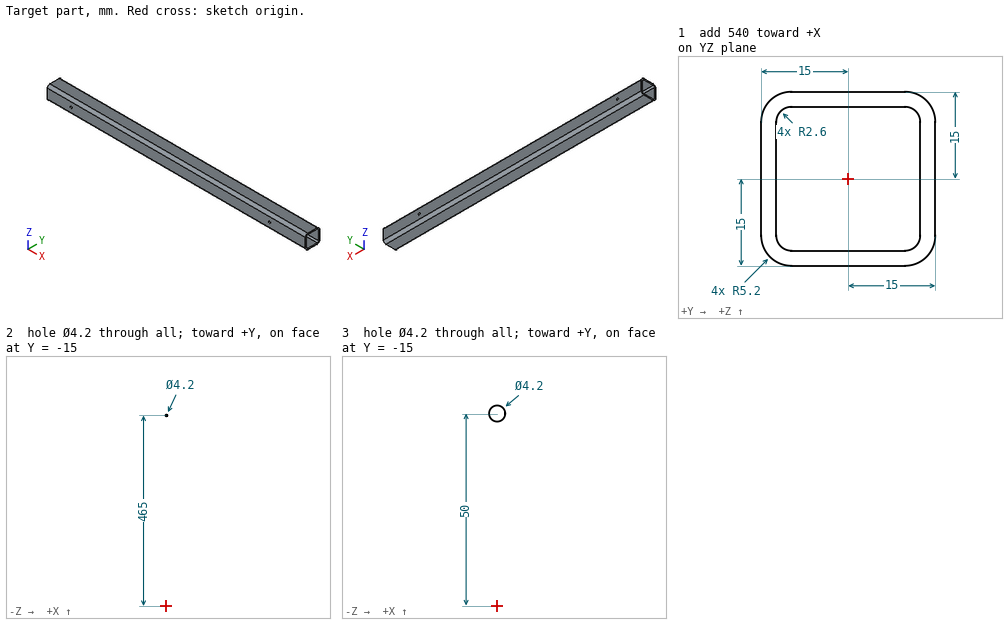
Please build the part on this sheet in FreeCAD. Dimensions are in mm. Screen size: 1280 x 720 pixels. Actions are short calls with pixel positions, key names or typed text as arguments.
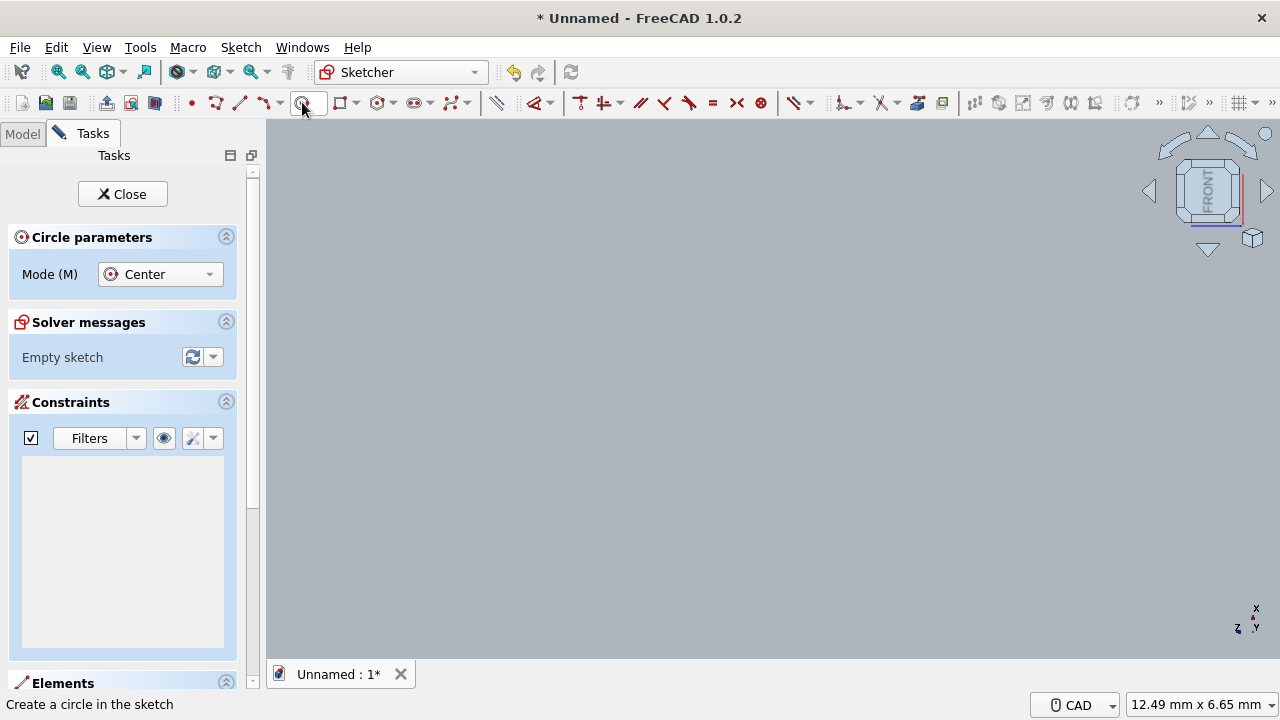
click(704, 388)
click(825, 268)
key(Escape)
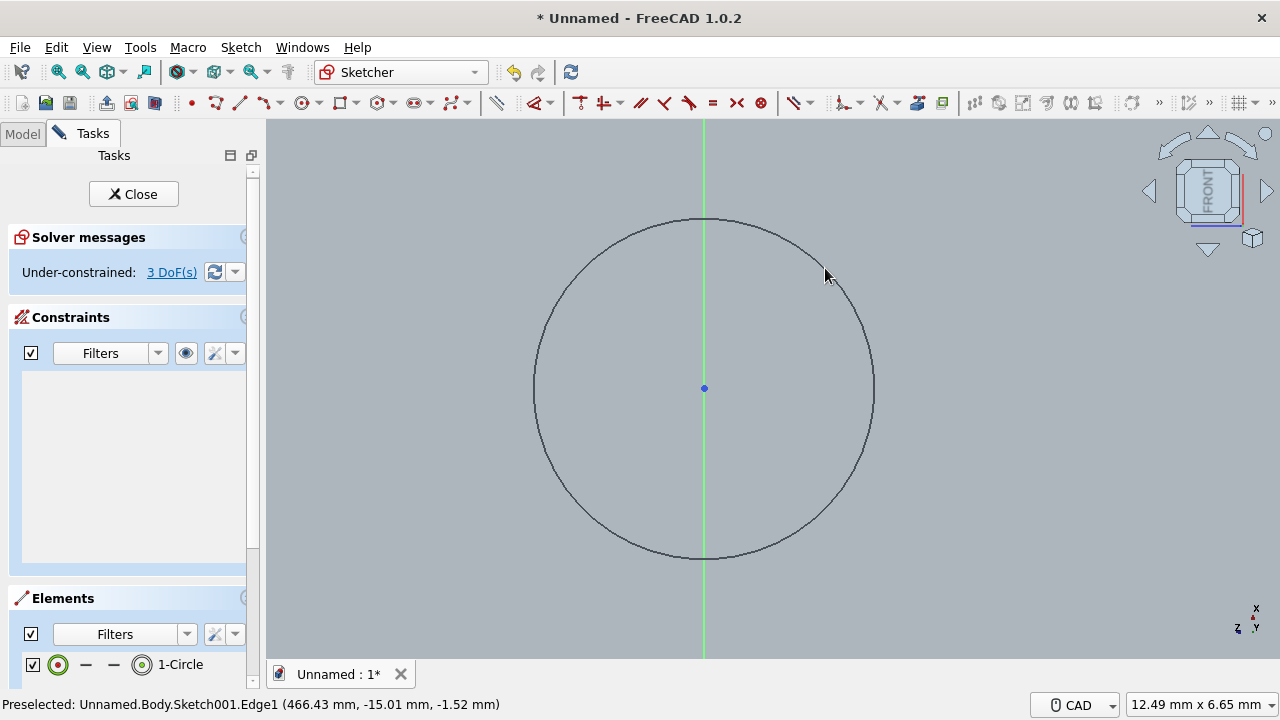
click(704, 389)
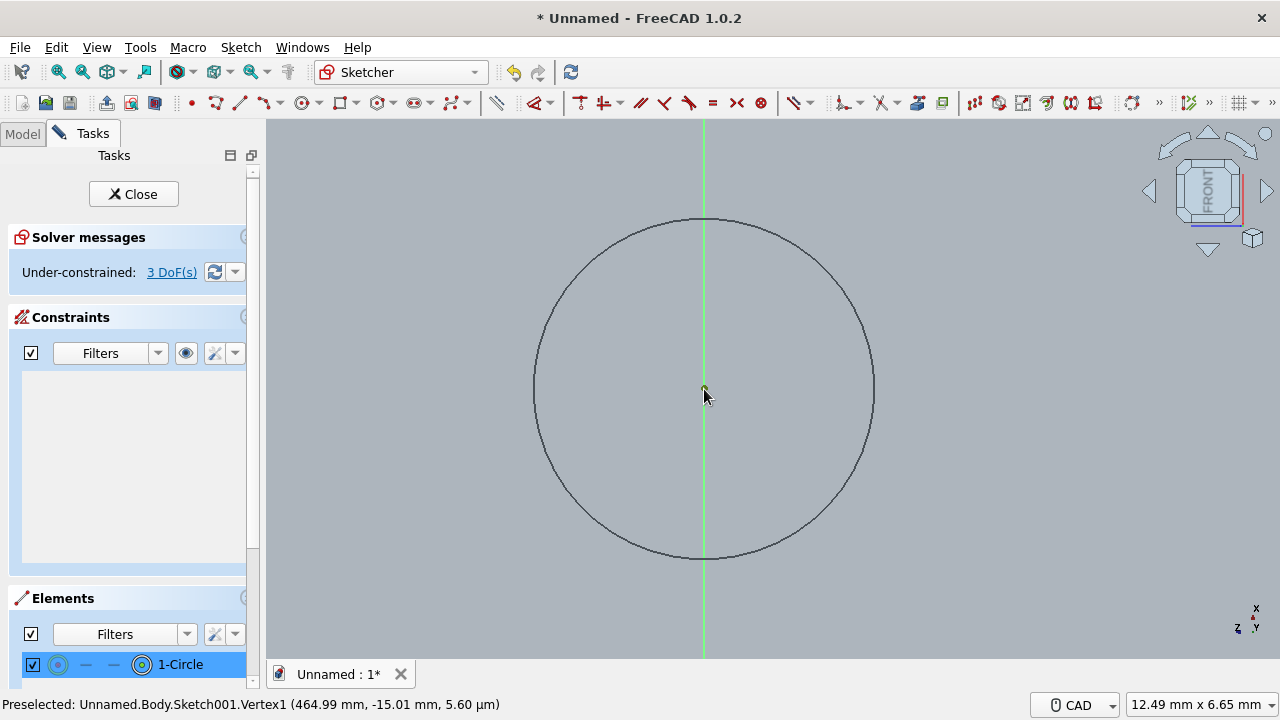
click(704, 596)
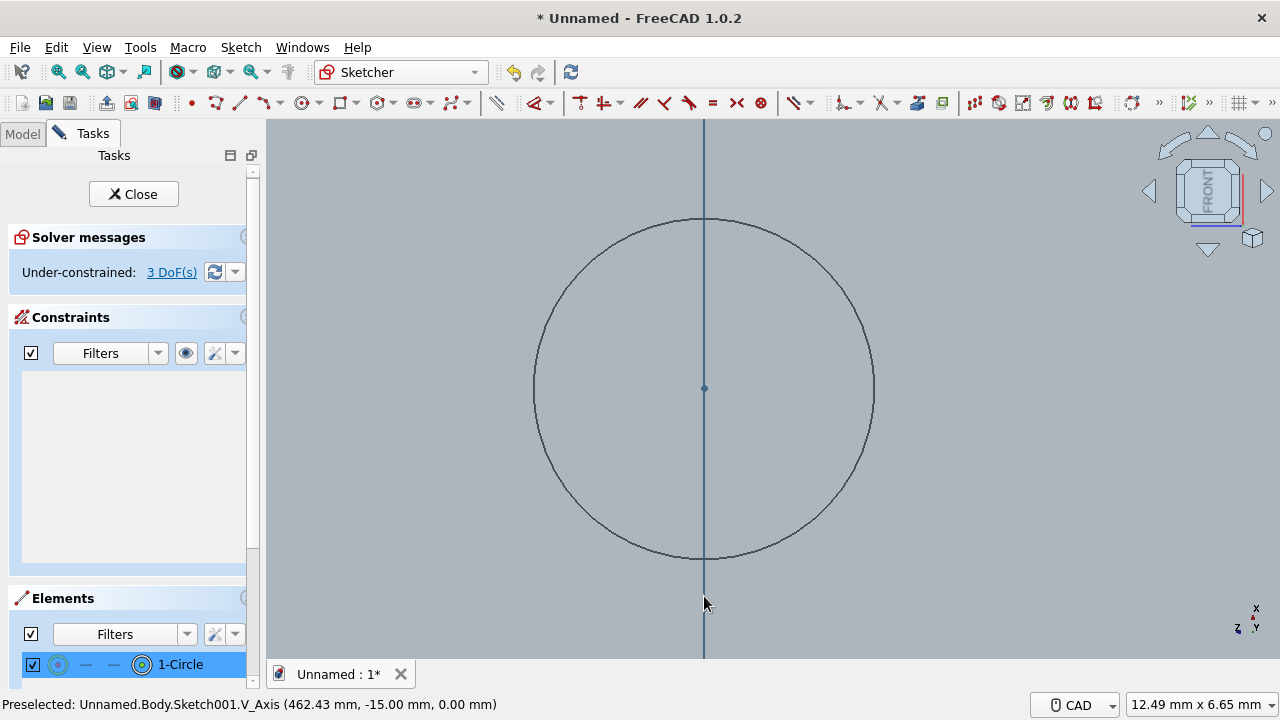
key(c)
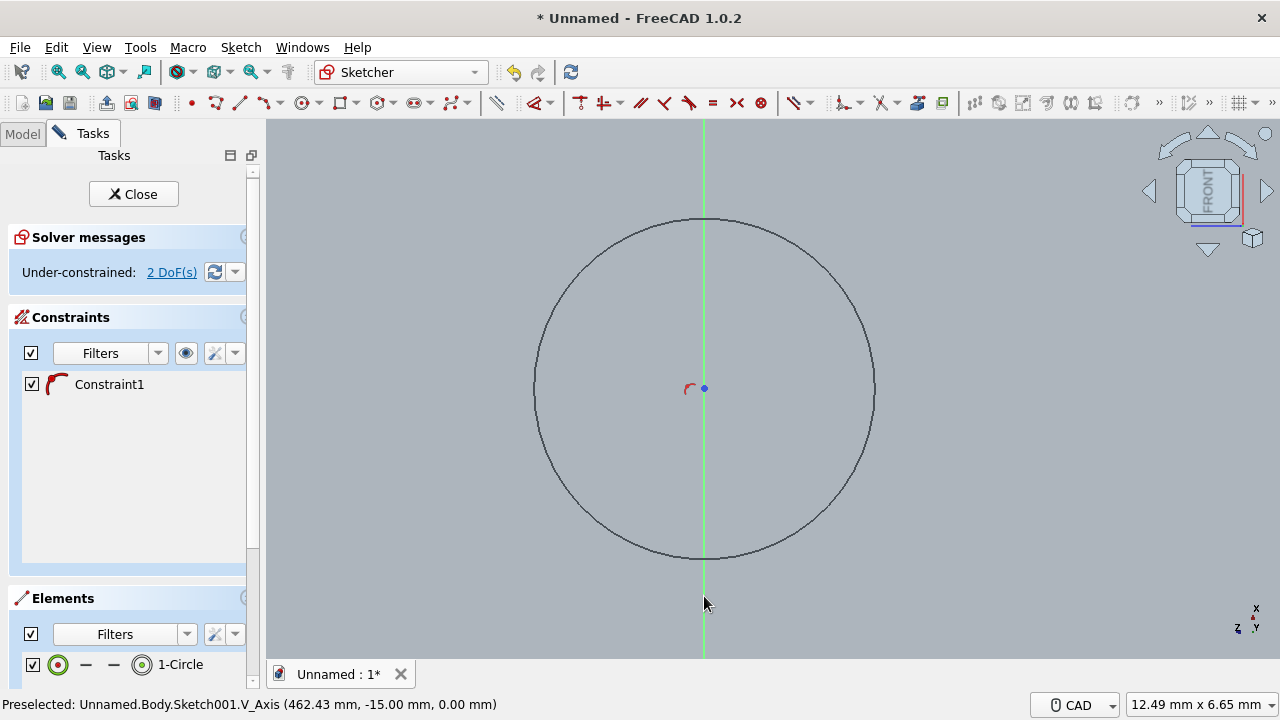
click(534, 104)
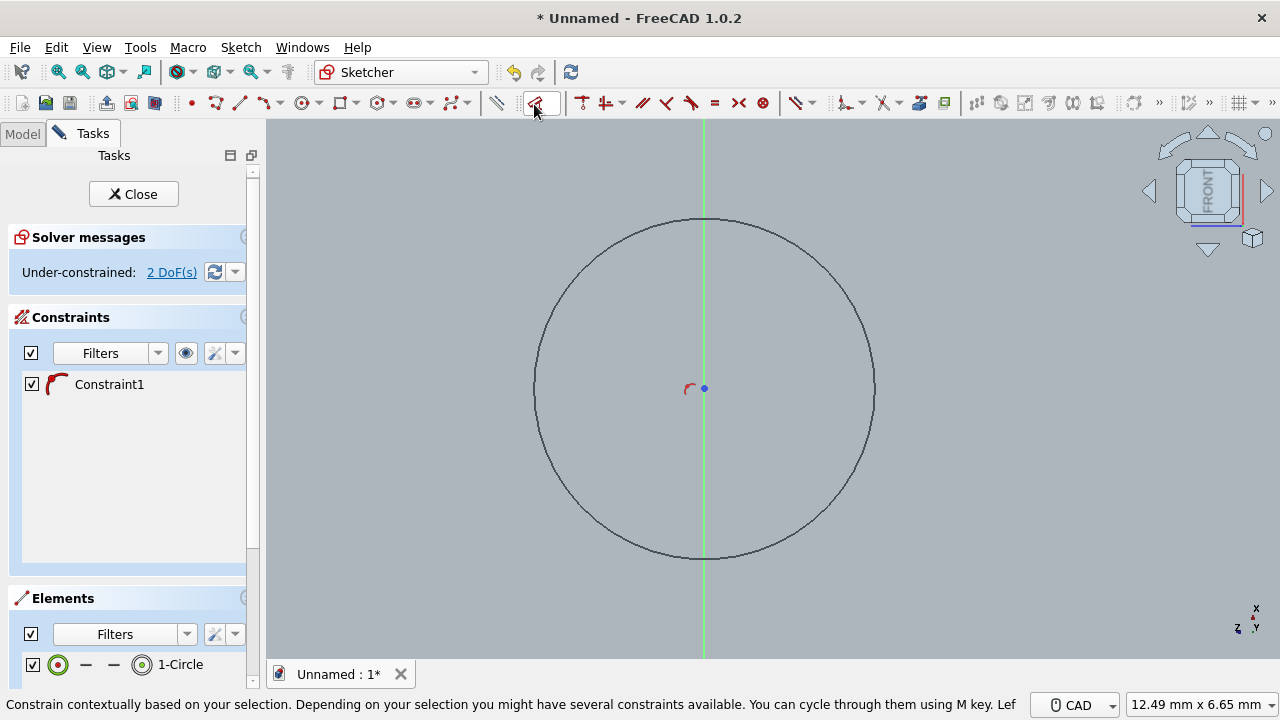
click(825, 268)
click(848, 245)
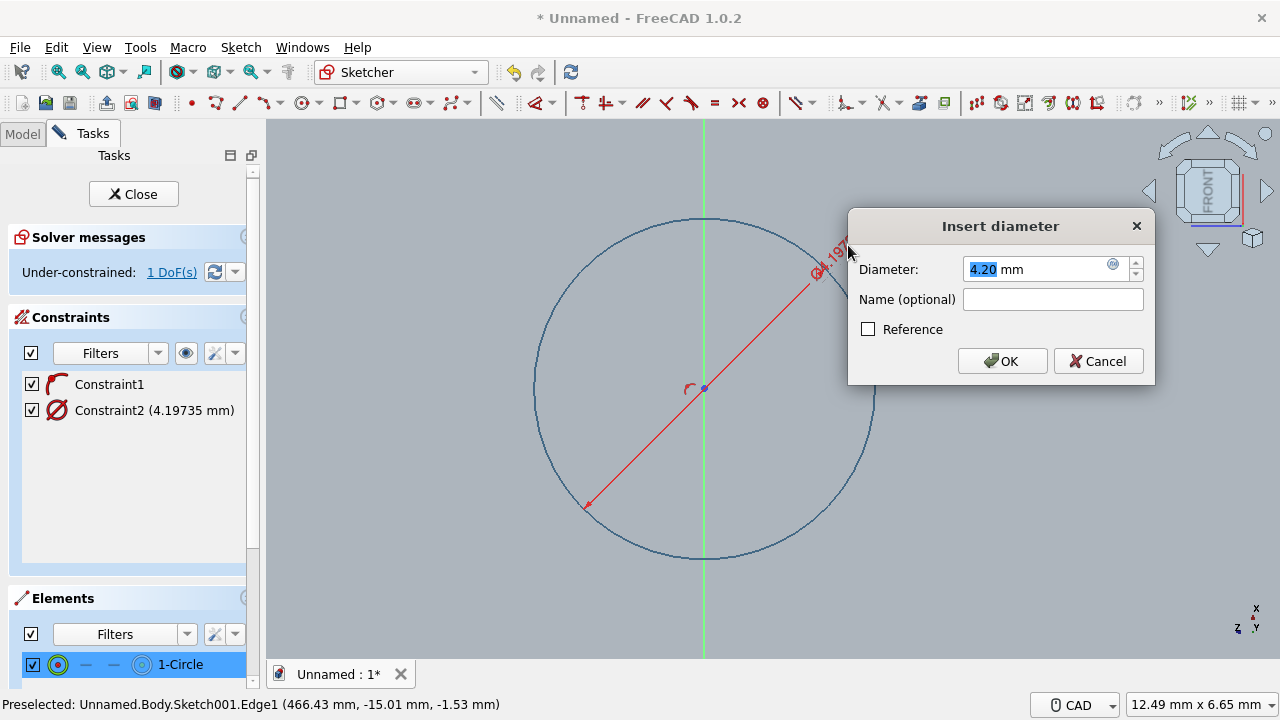
text(4.2)
key(Return)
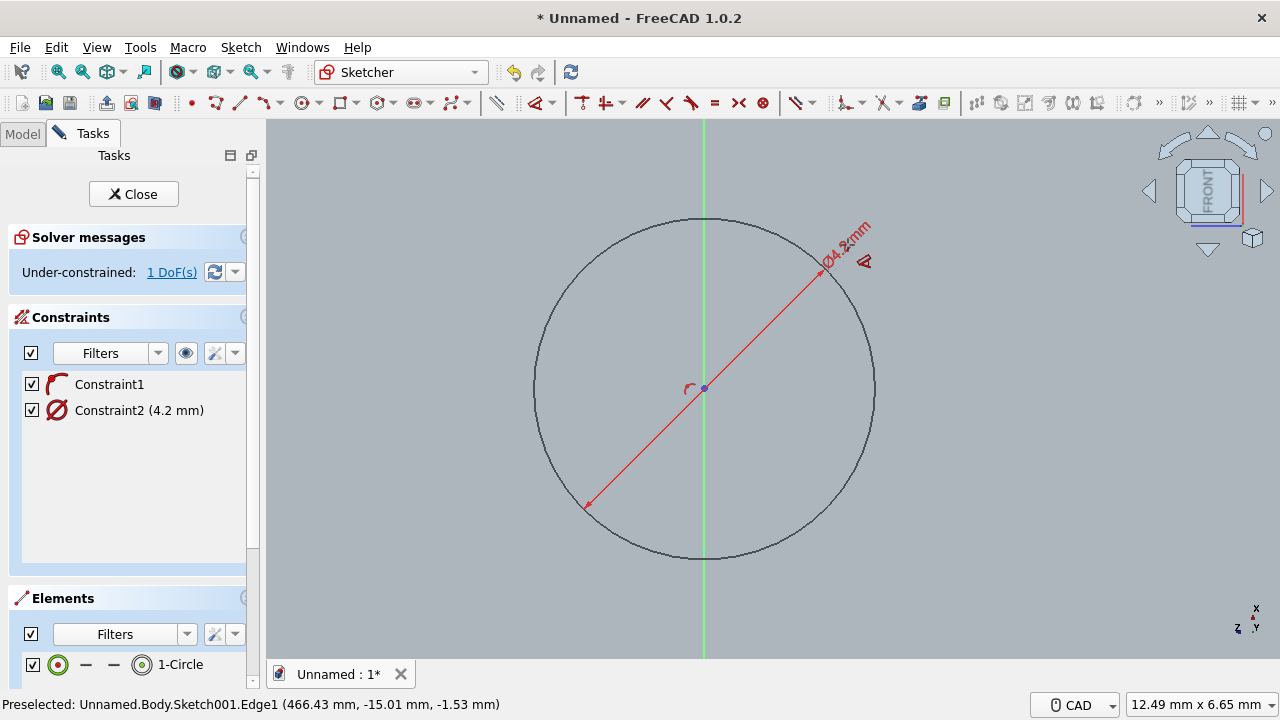
click(704, 389)
click(738, 510)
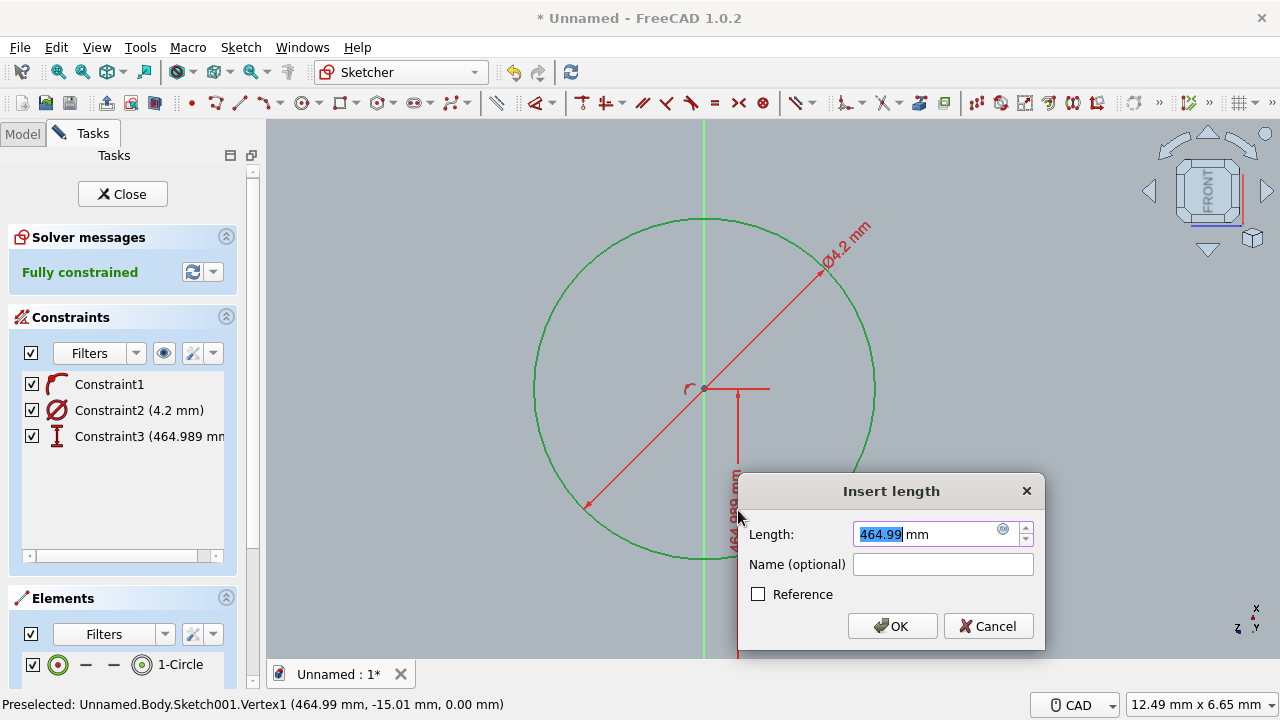
text(465)
key(Return)
key(Escape)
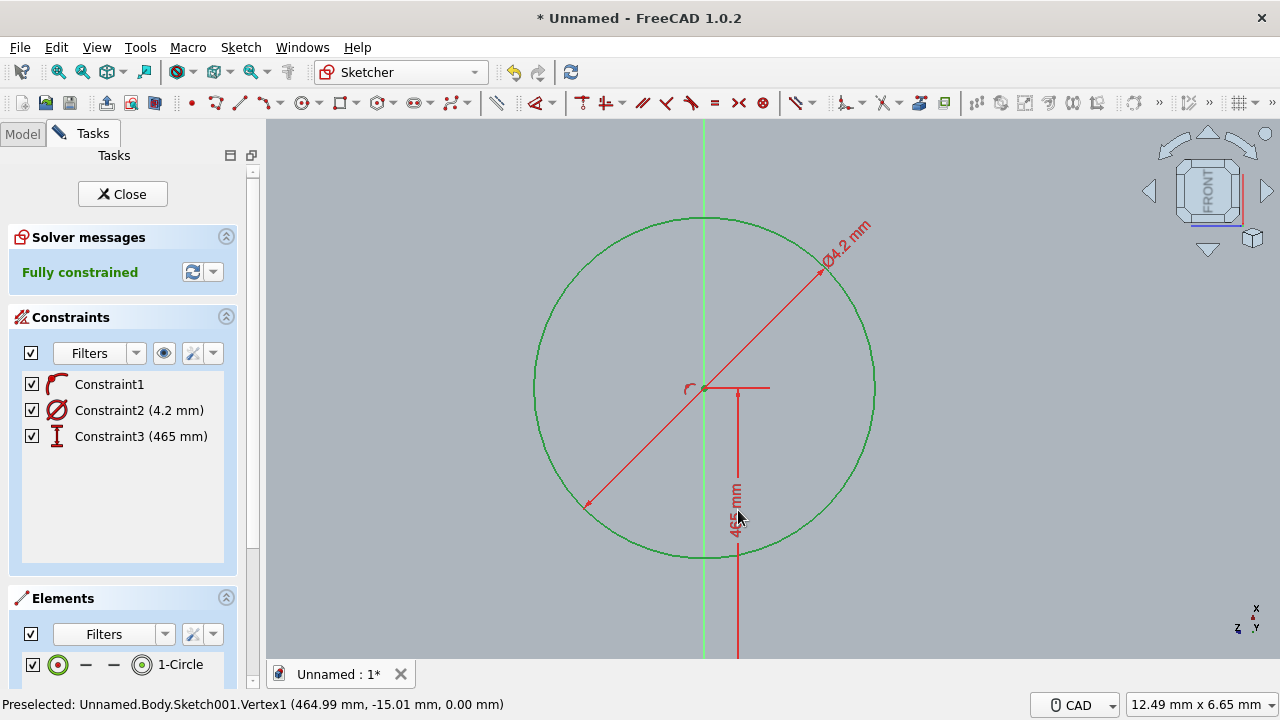
click(123, 194)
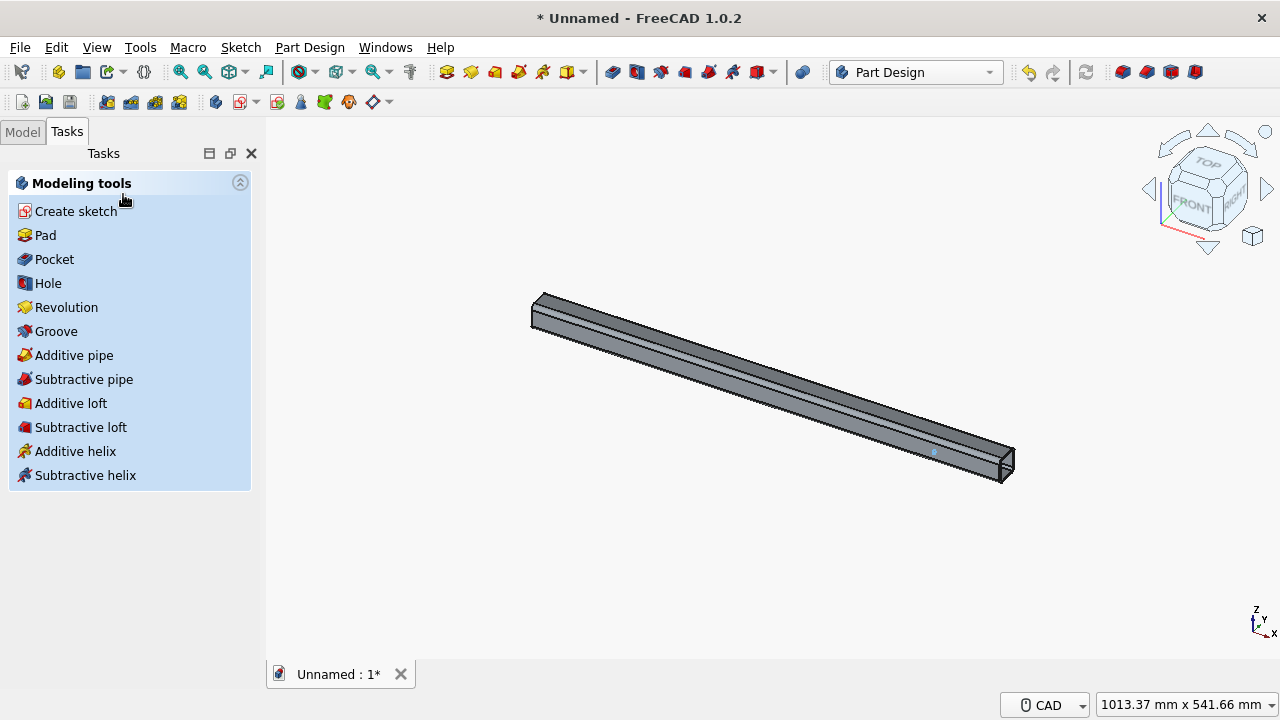
click(638, 72)